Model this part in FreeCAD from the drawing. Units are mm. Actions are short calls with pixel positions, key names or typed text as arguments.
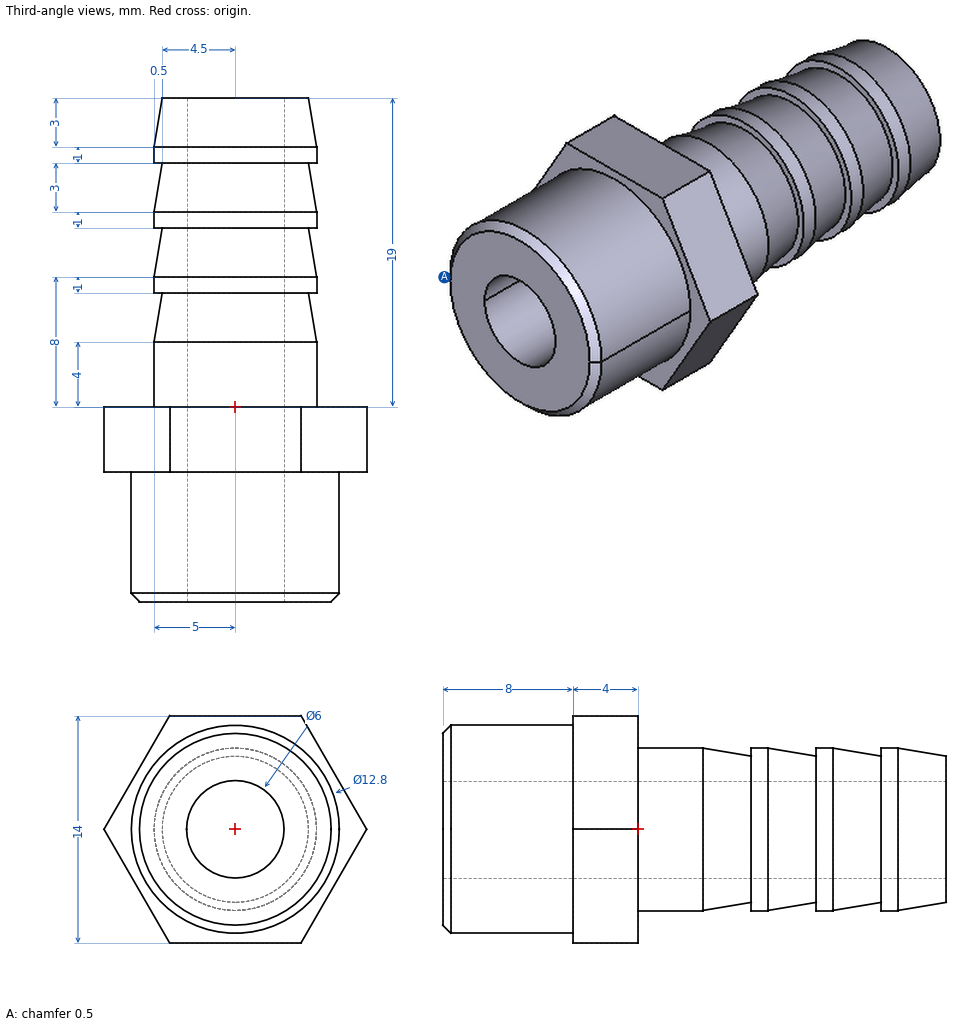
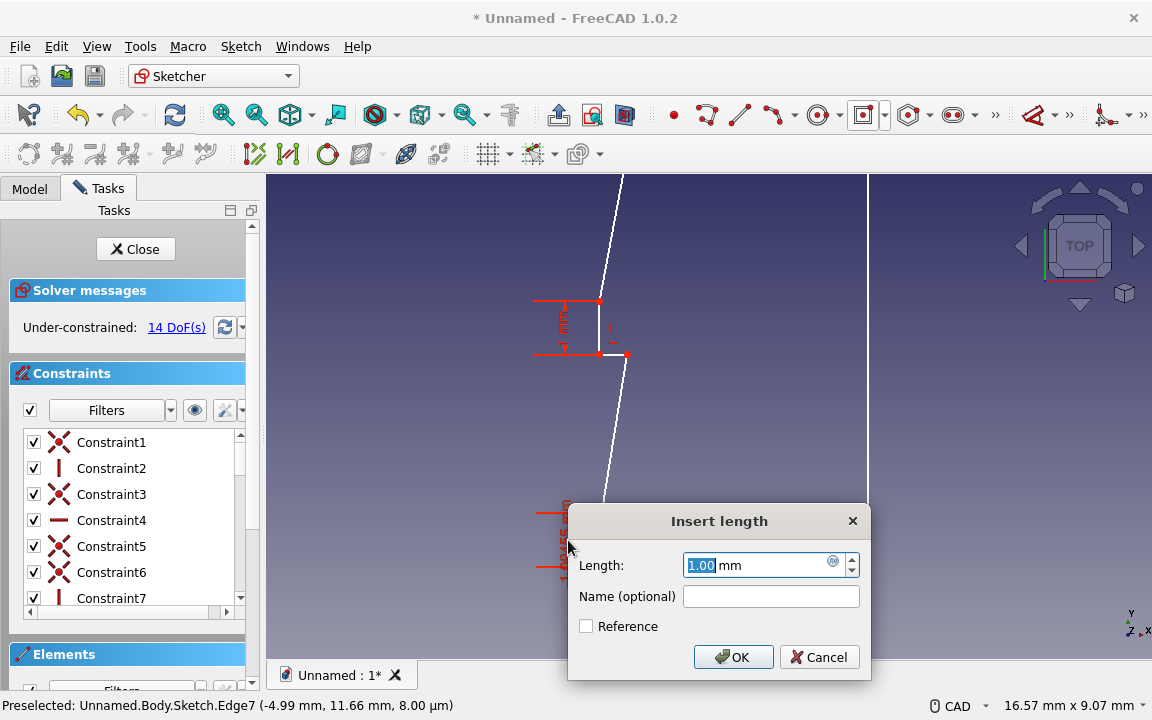
text(1)
key(Return)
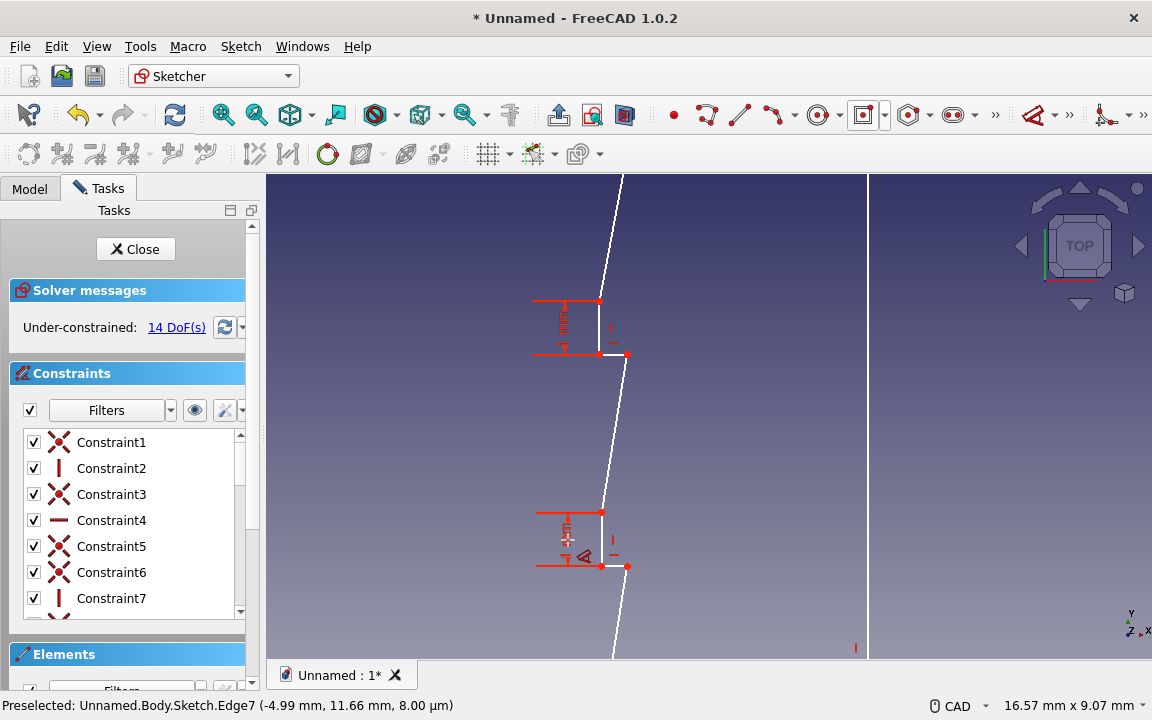
scroll(600, 318, down, 6)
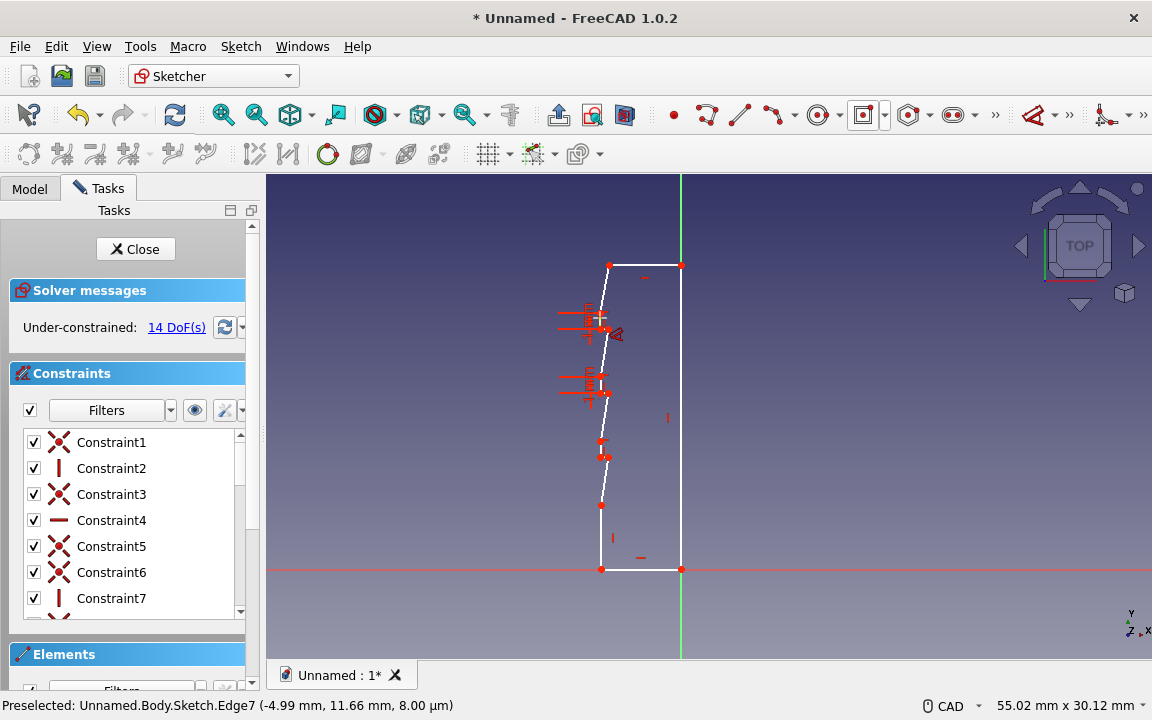
scroll(601, 446, up, 6)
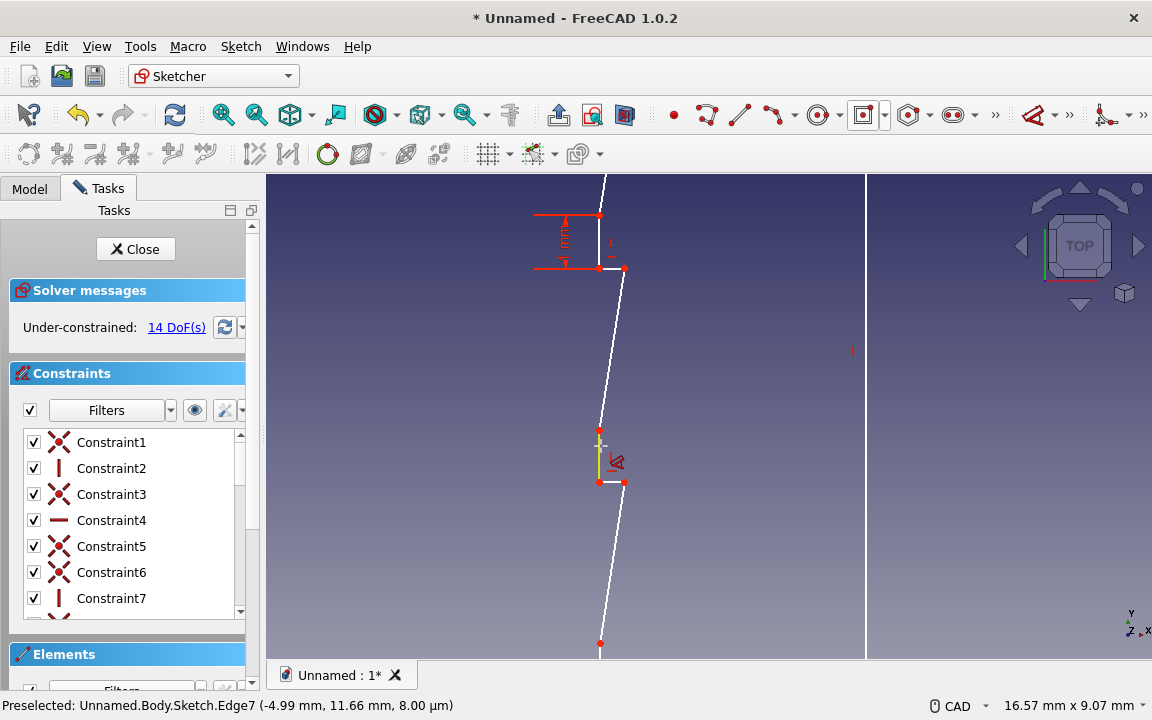
click(599, 446)
click(565, 456)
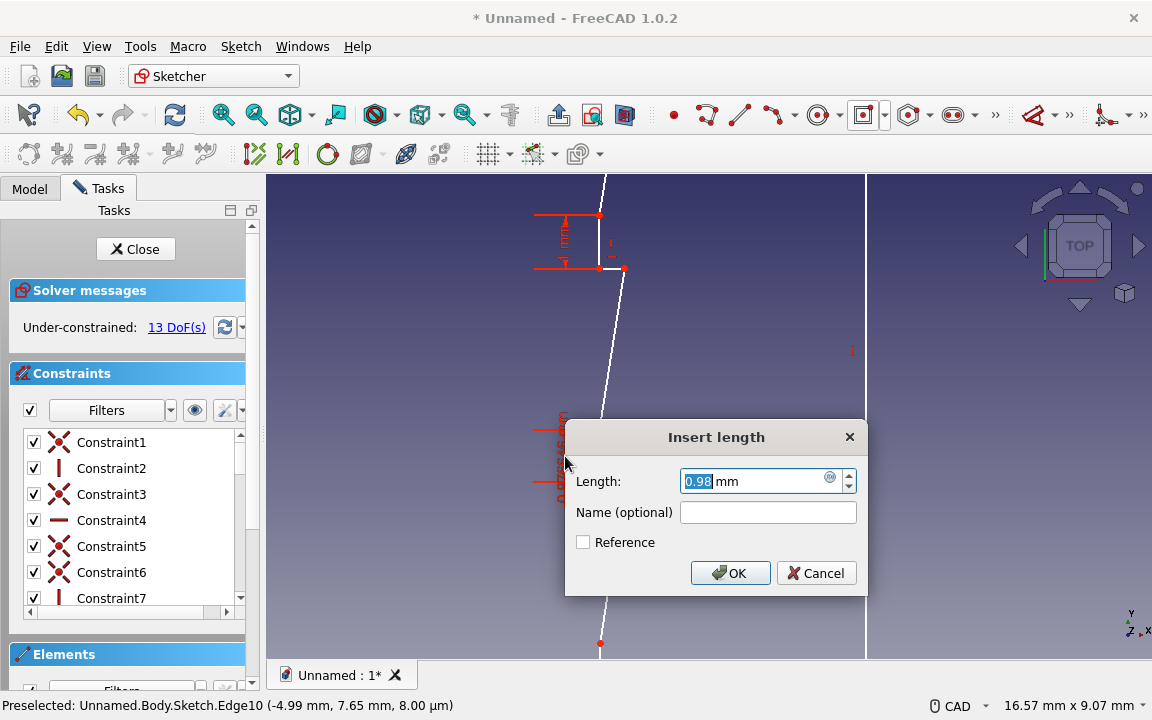
text(1)
key(Return)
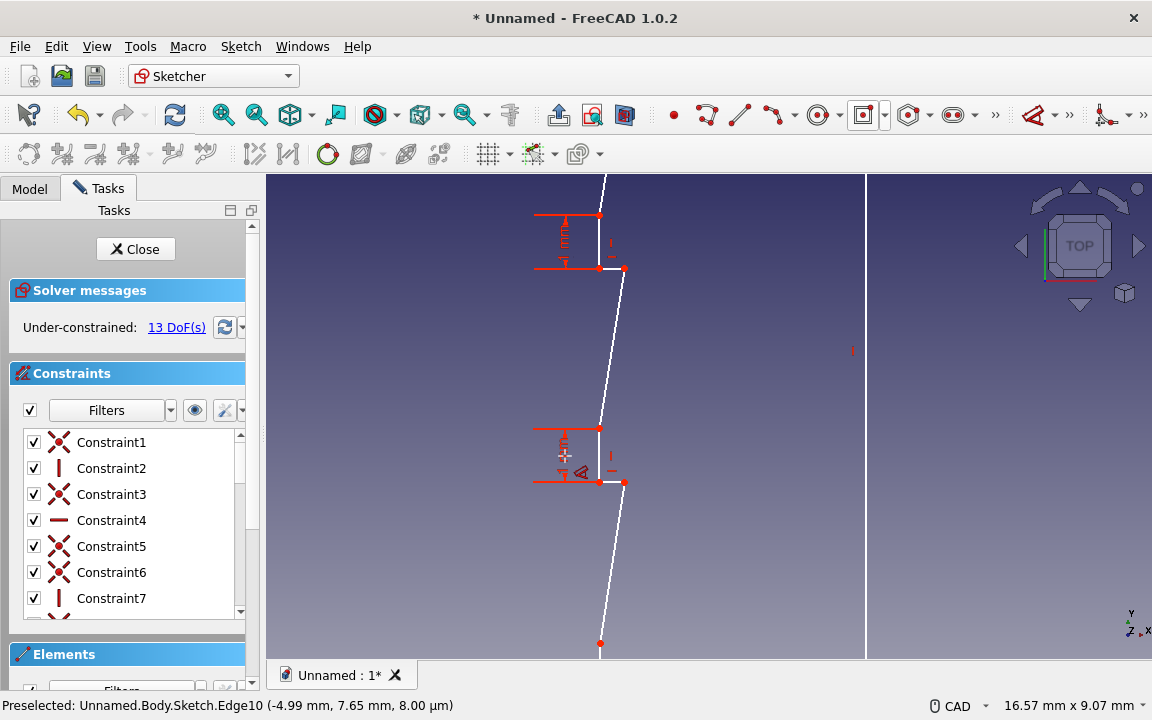
scroll(601, 446, down, 6)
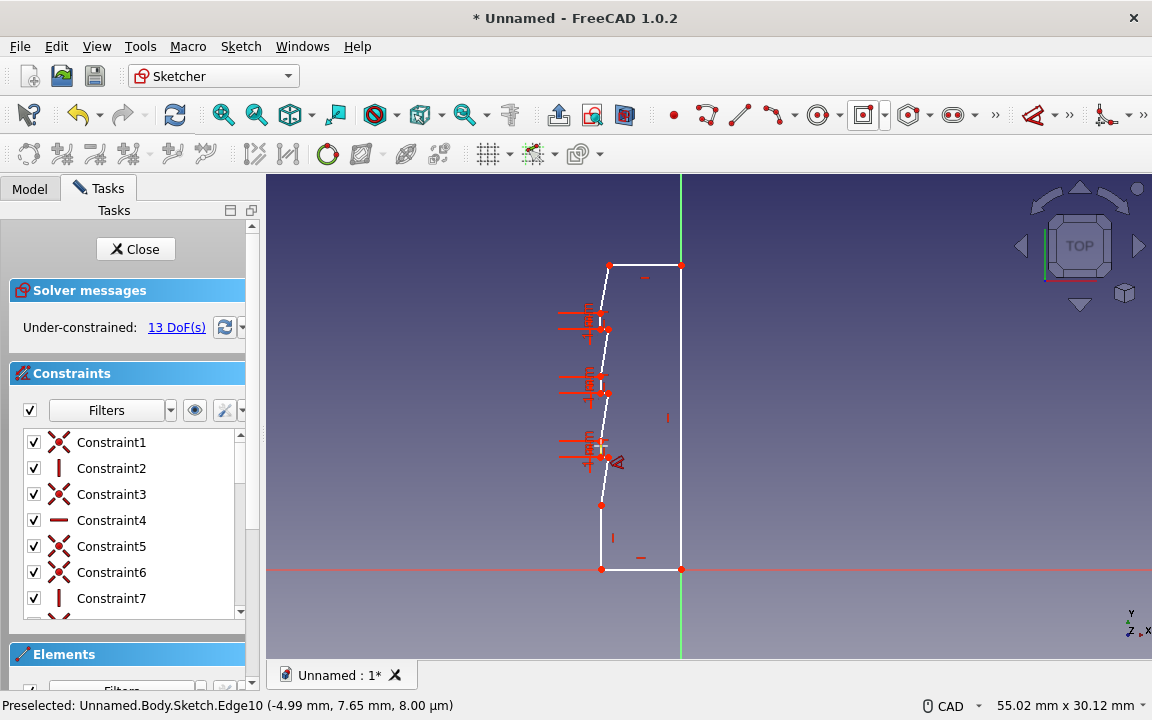
click(601, 525)
click(567, 538)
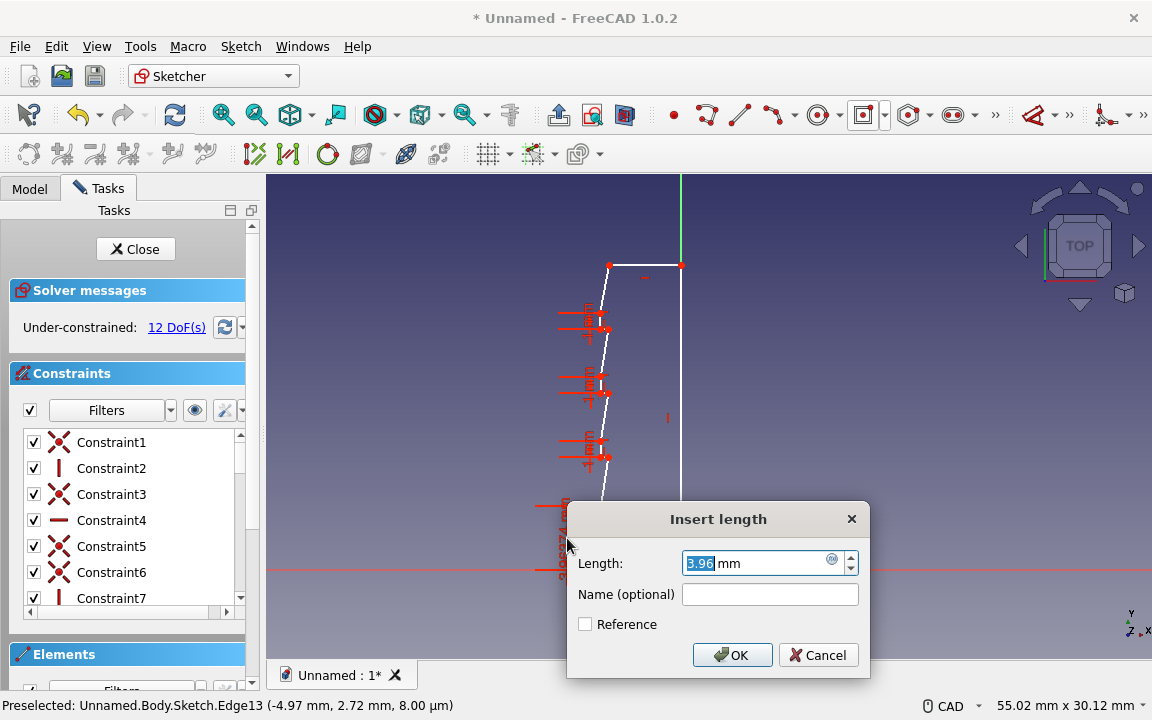
text(4)
key(Return)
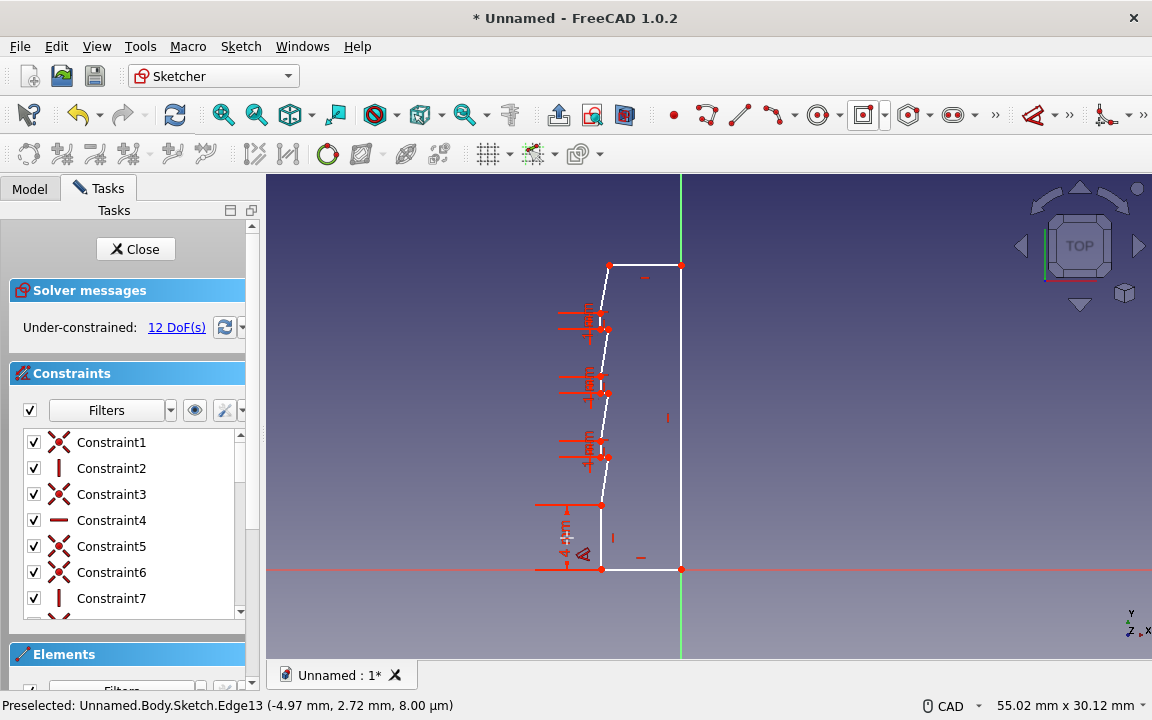
click(625, 570)
click(641, 604)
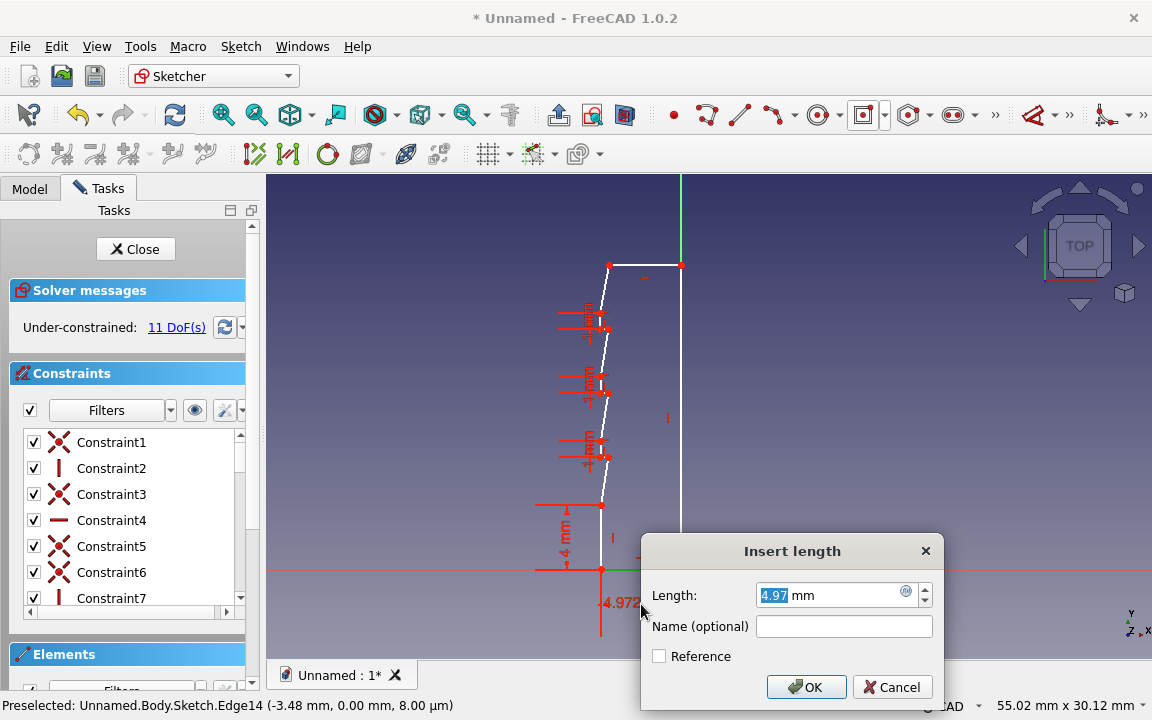
text(5)
key(Return)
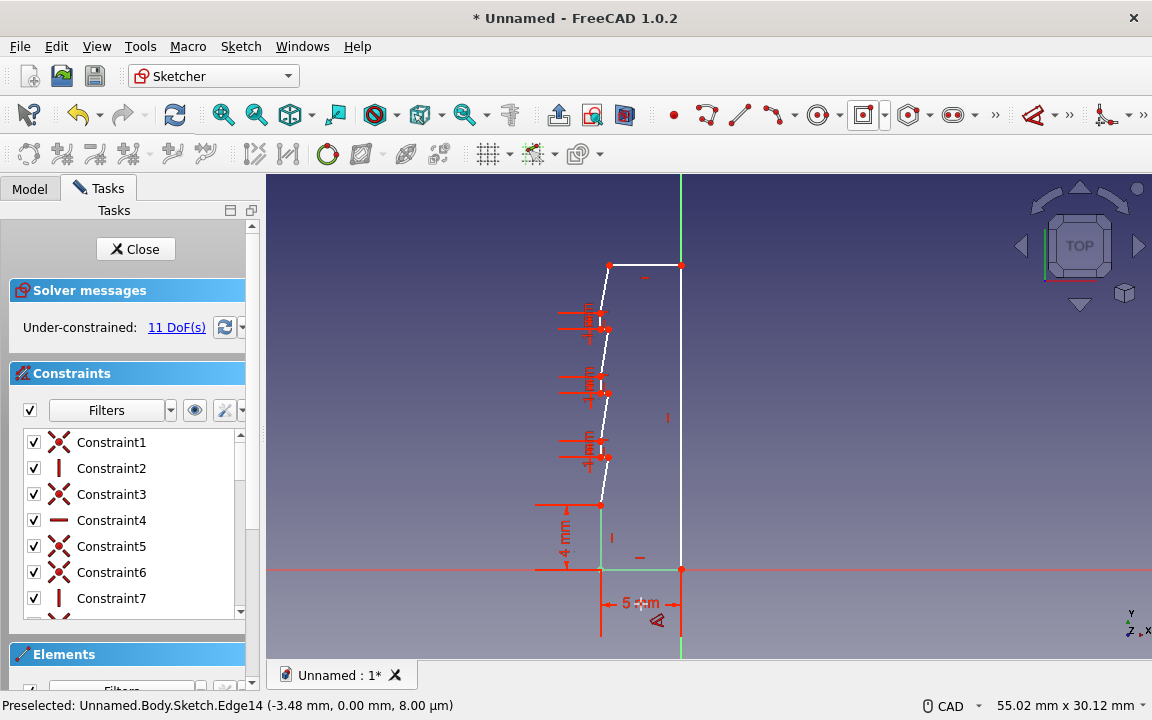
click(681, 478)
click(715, 418)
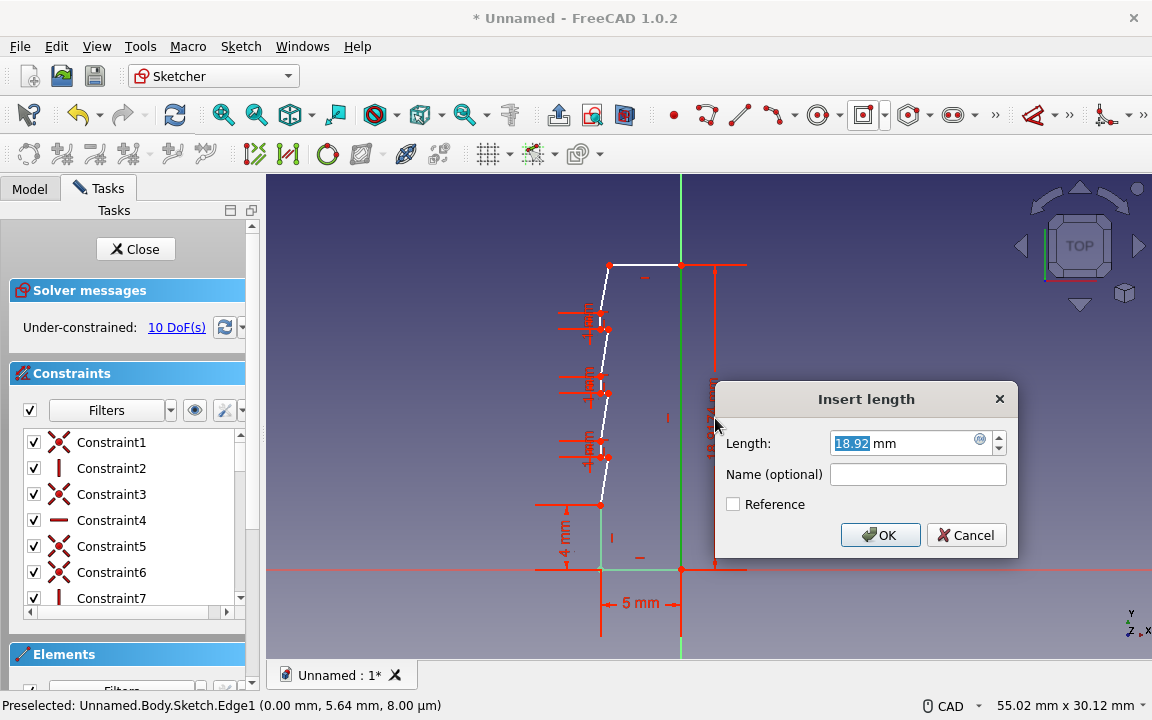
text(19)
key(Return)